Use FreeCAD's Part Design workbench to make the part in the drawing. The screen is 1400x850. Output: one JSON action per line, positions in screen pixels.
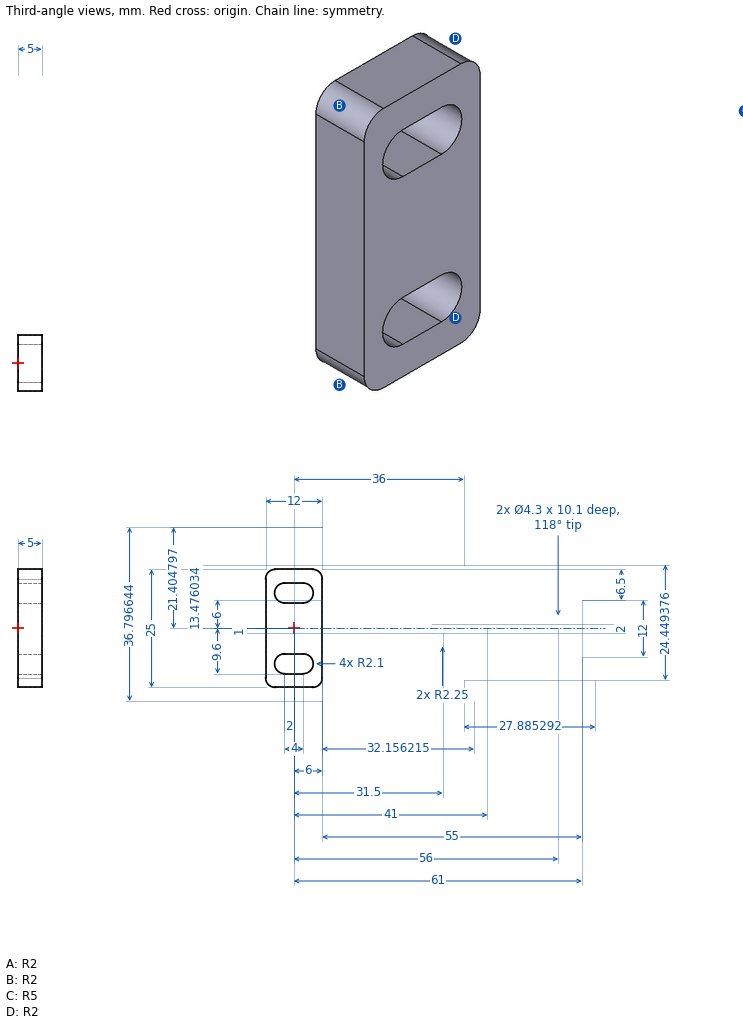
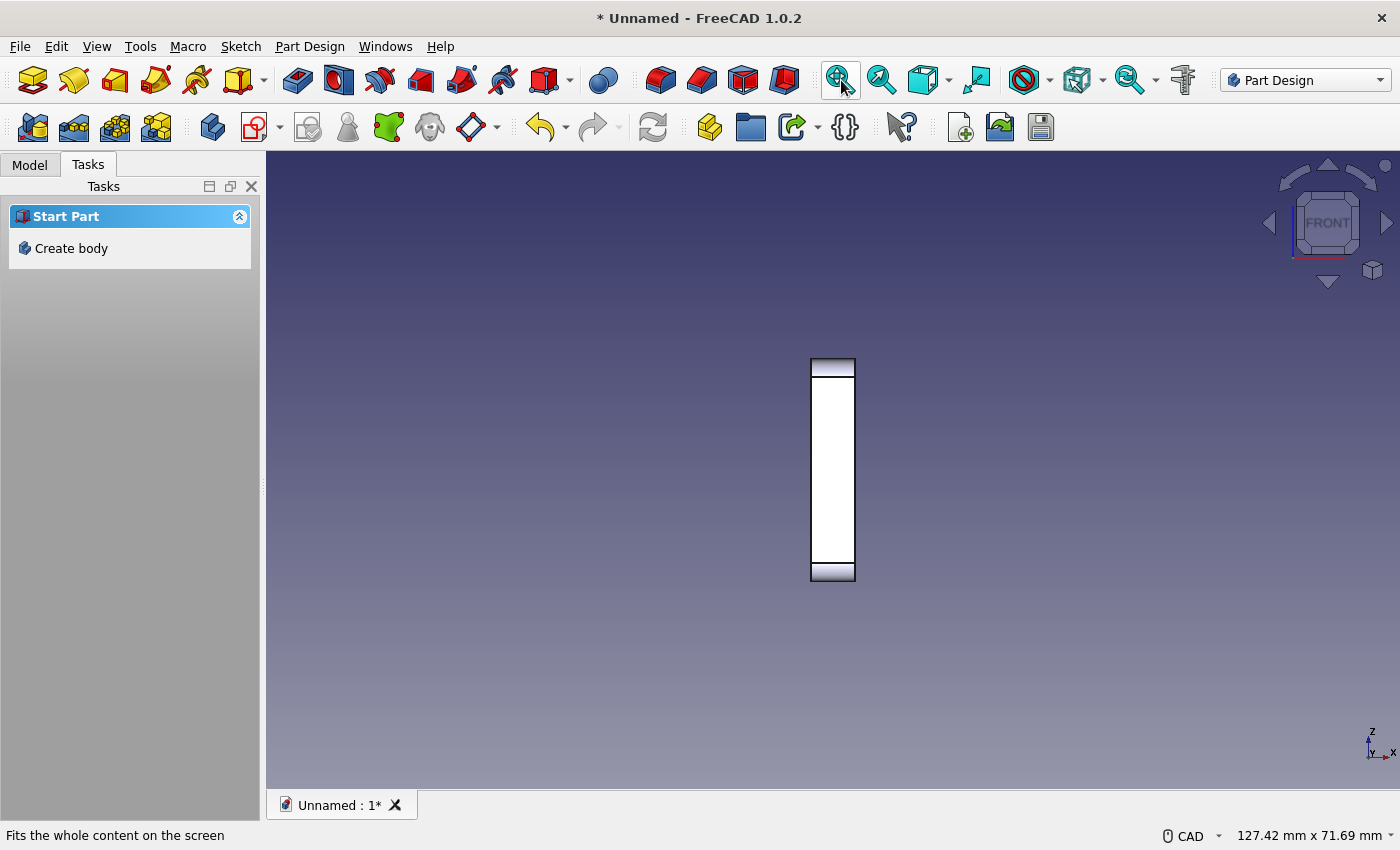
{"action": "key", "text": "0"}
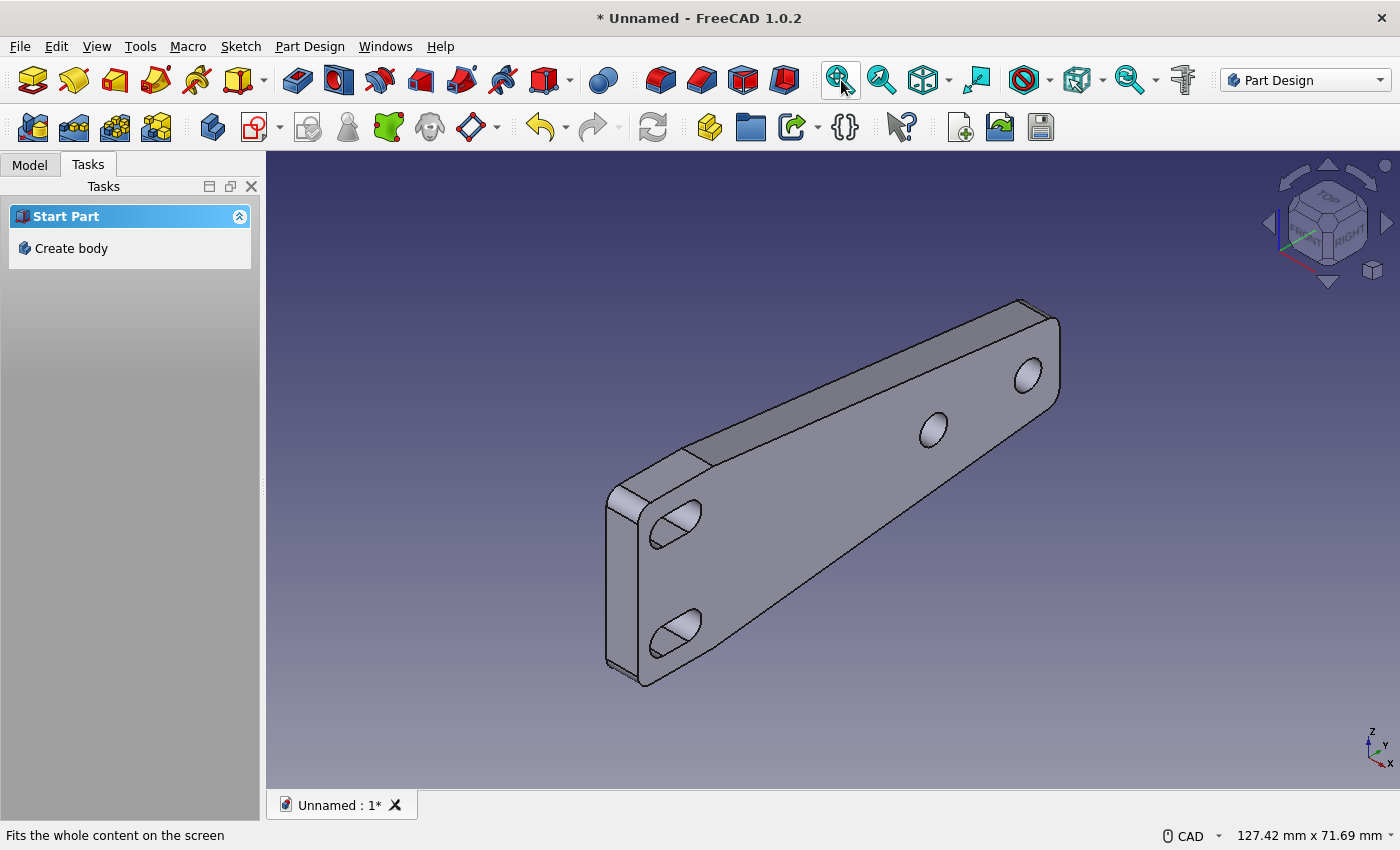
{"action": "left_click", "coordinate": [788, 513]}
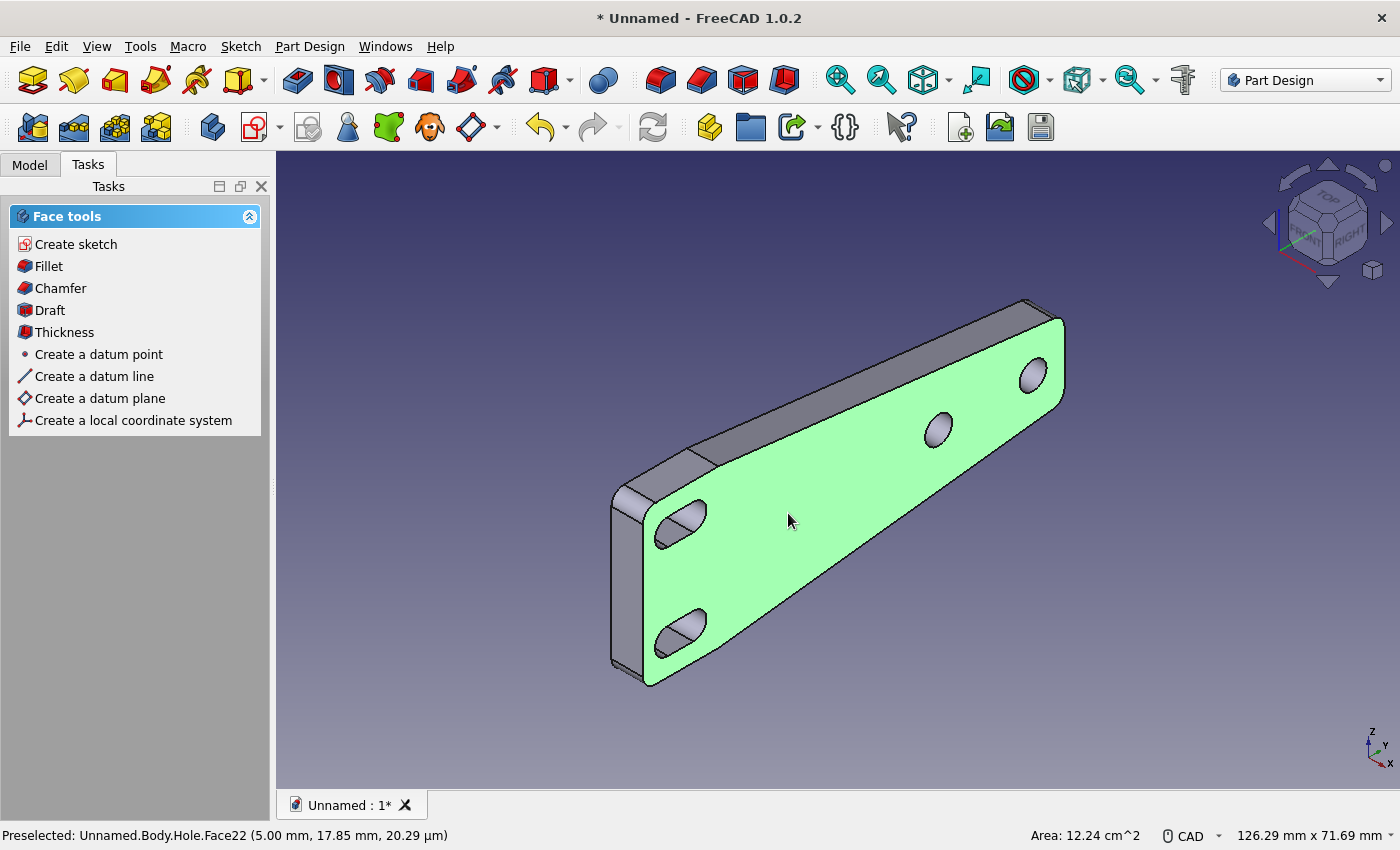
{"action": "left_click", "coordinate": [254, 128]}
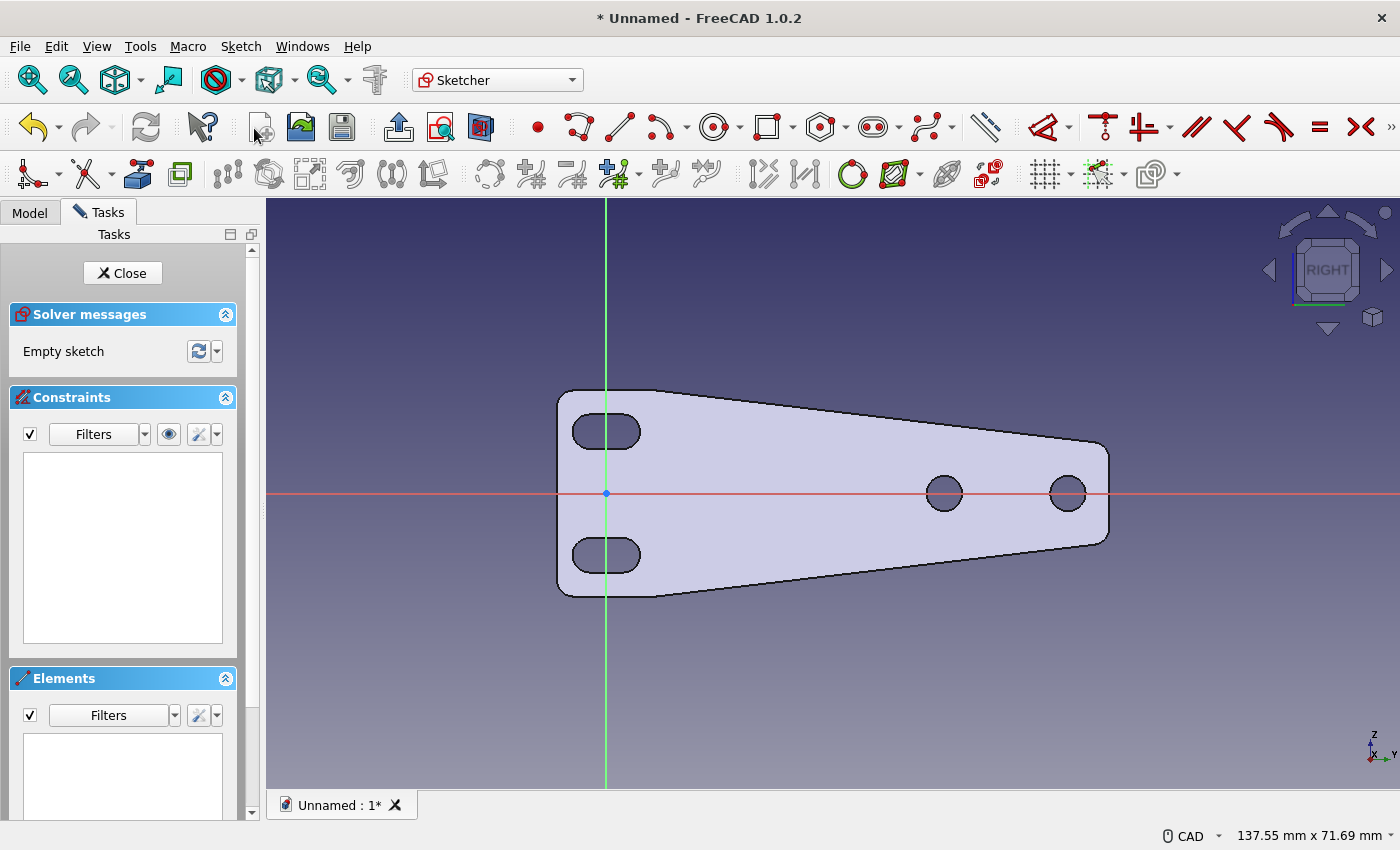
{"action": "left_click", "coordinate": [766, 128]}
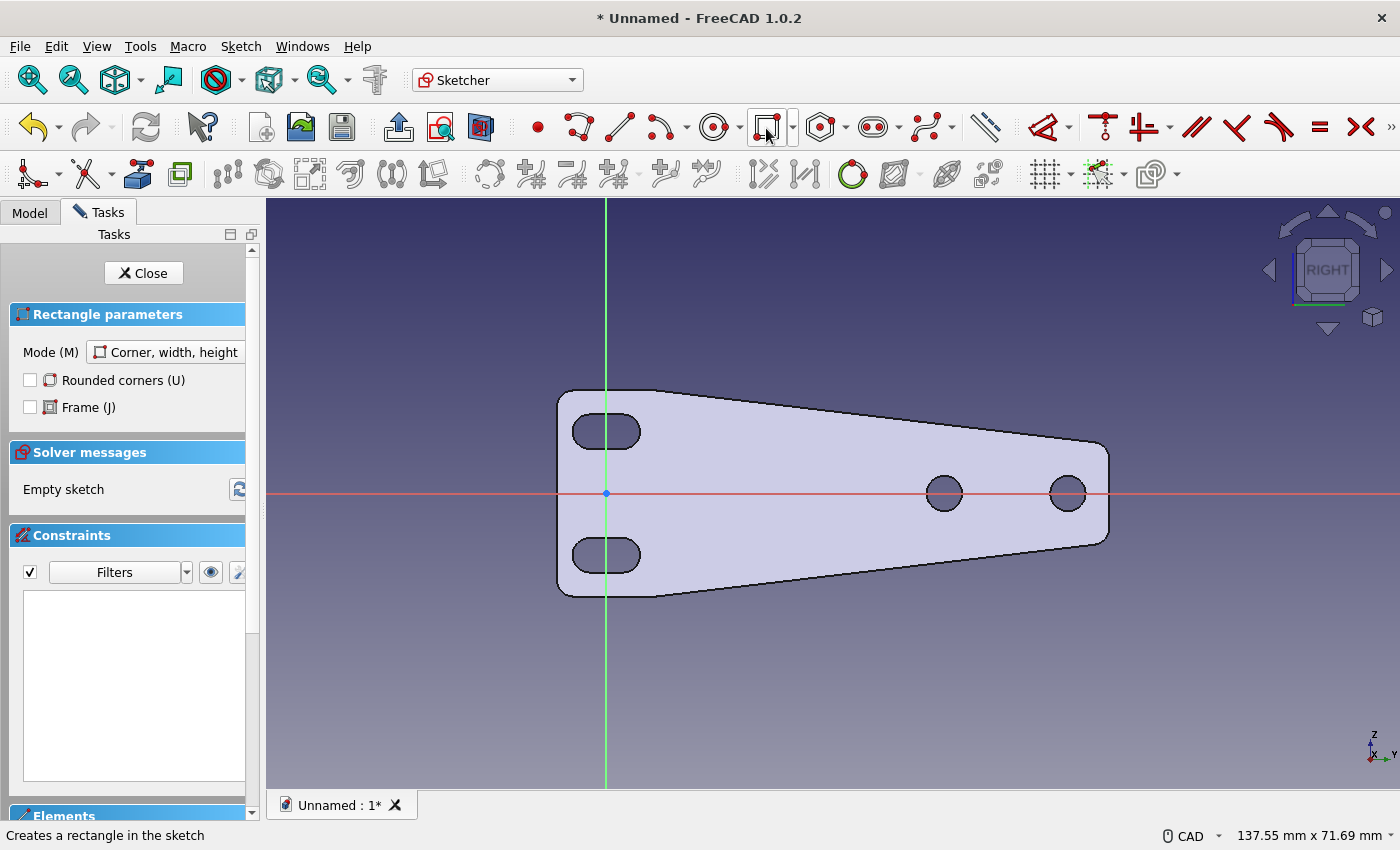
{"action": "left_click", "coordinate": [903, 382]}
{"action": "left_click", "coordinate": [1133, 584]}
{"action": "key", "text": "Escape"}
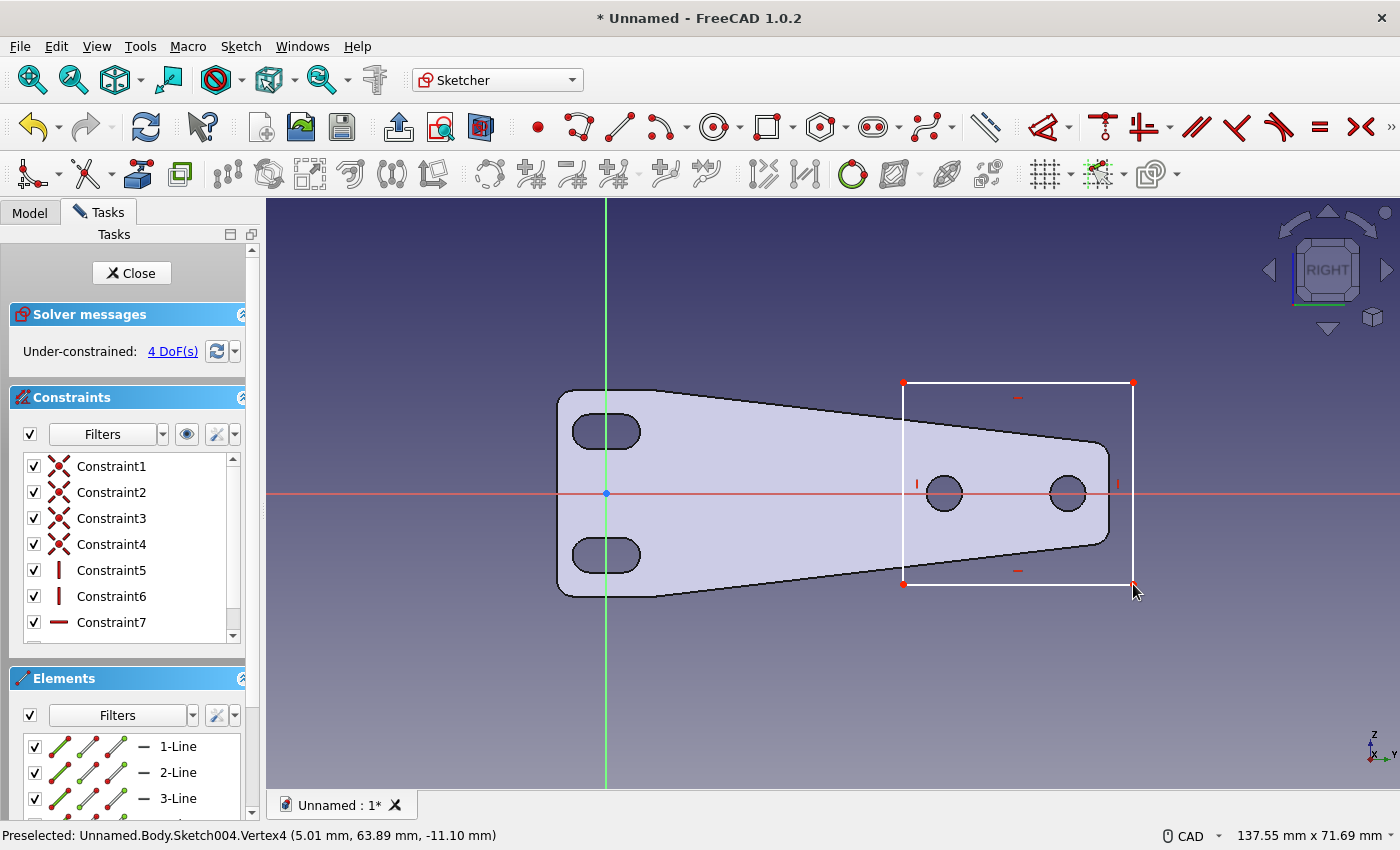
{"action": "left_click", "coordinate": [1042, 128]}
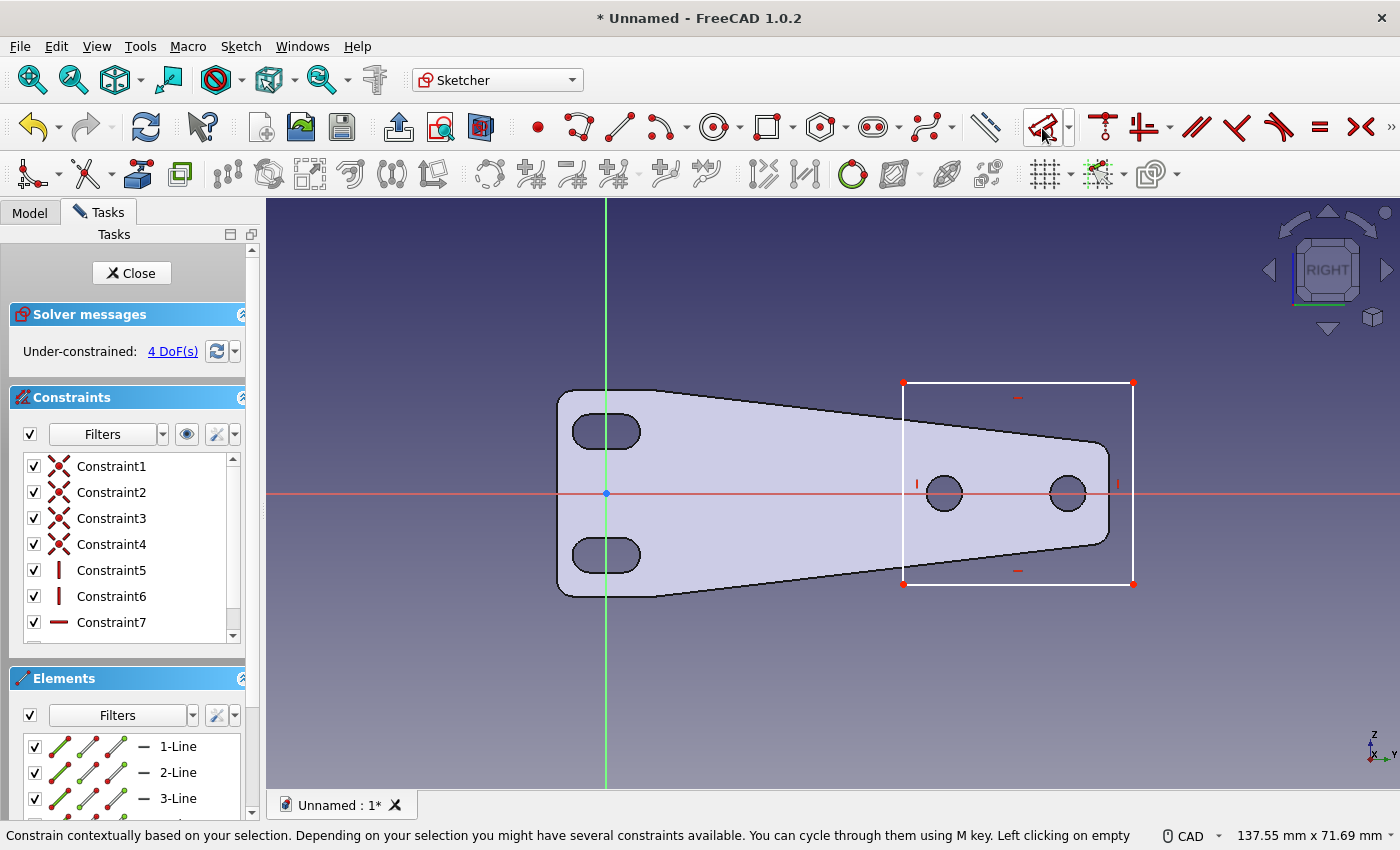
{"action": "left_click", "coordinate": [903, 383]}
{"action": "left_click", "coordinate": [755, 349]}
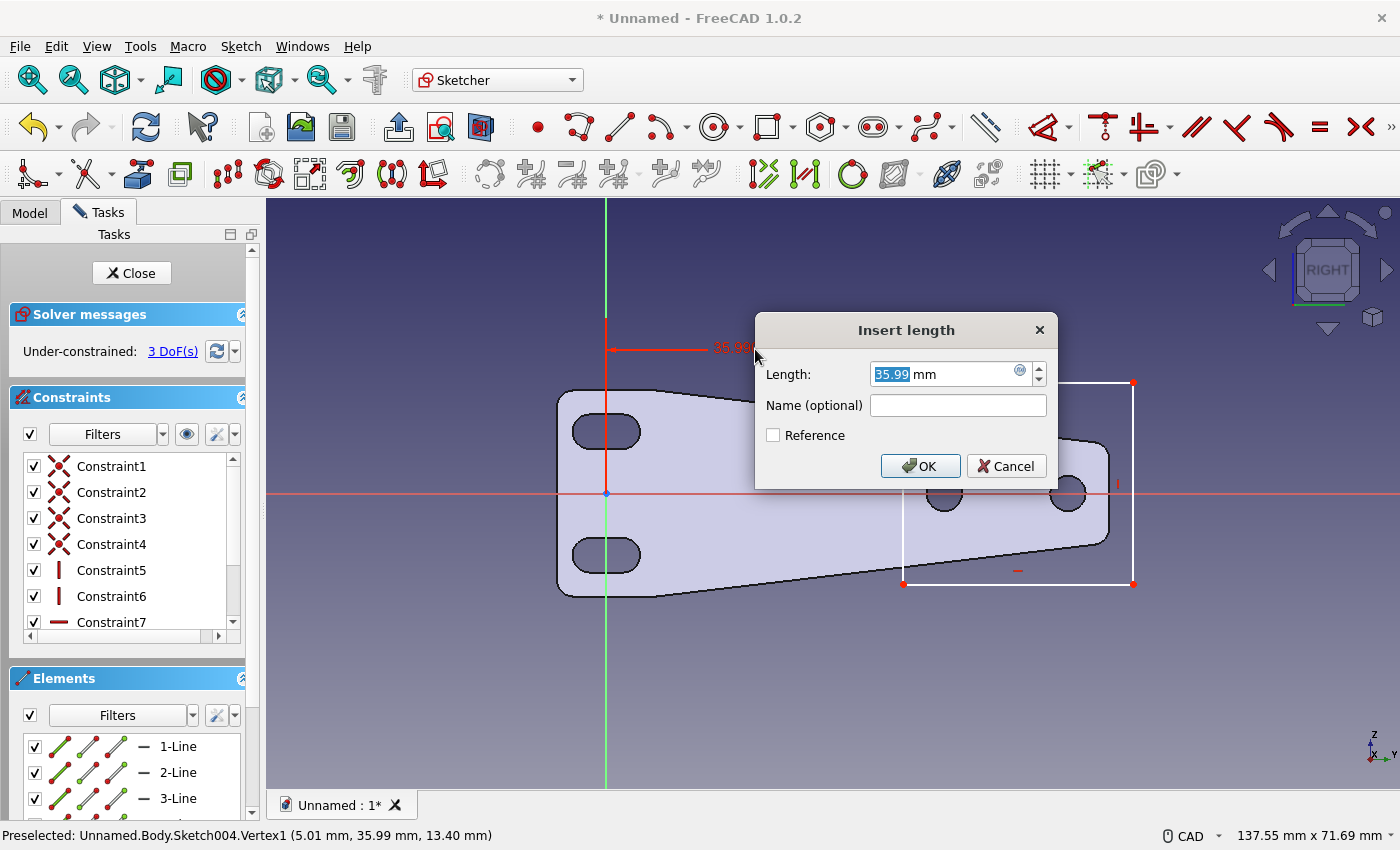
{"action": "type", "text": "36"}
{"action": "key", "text": "Return"}